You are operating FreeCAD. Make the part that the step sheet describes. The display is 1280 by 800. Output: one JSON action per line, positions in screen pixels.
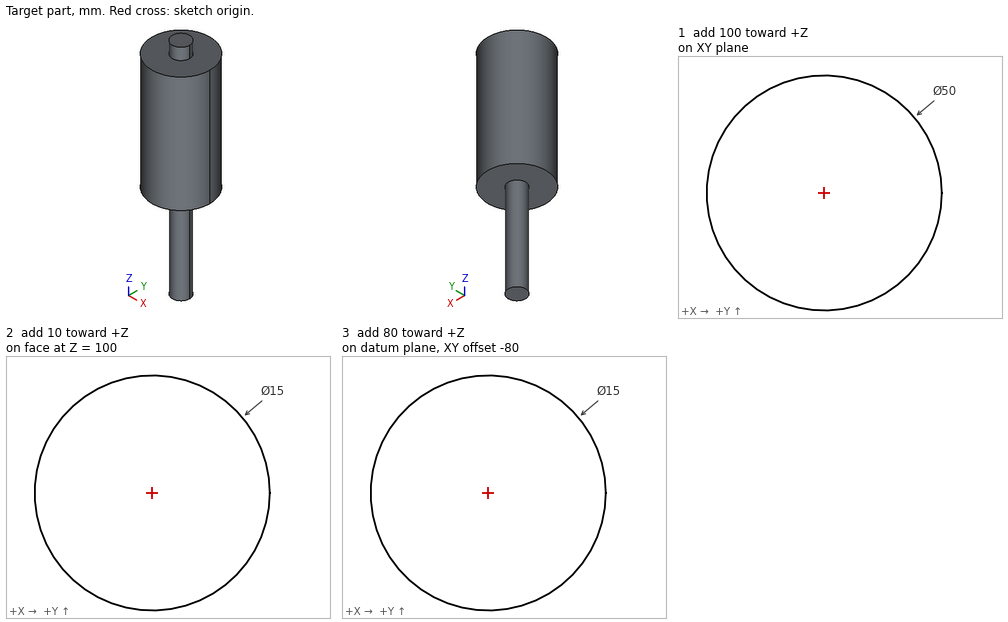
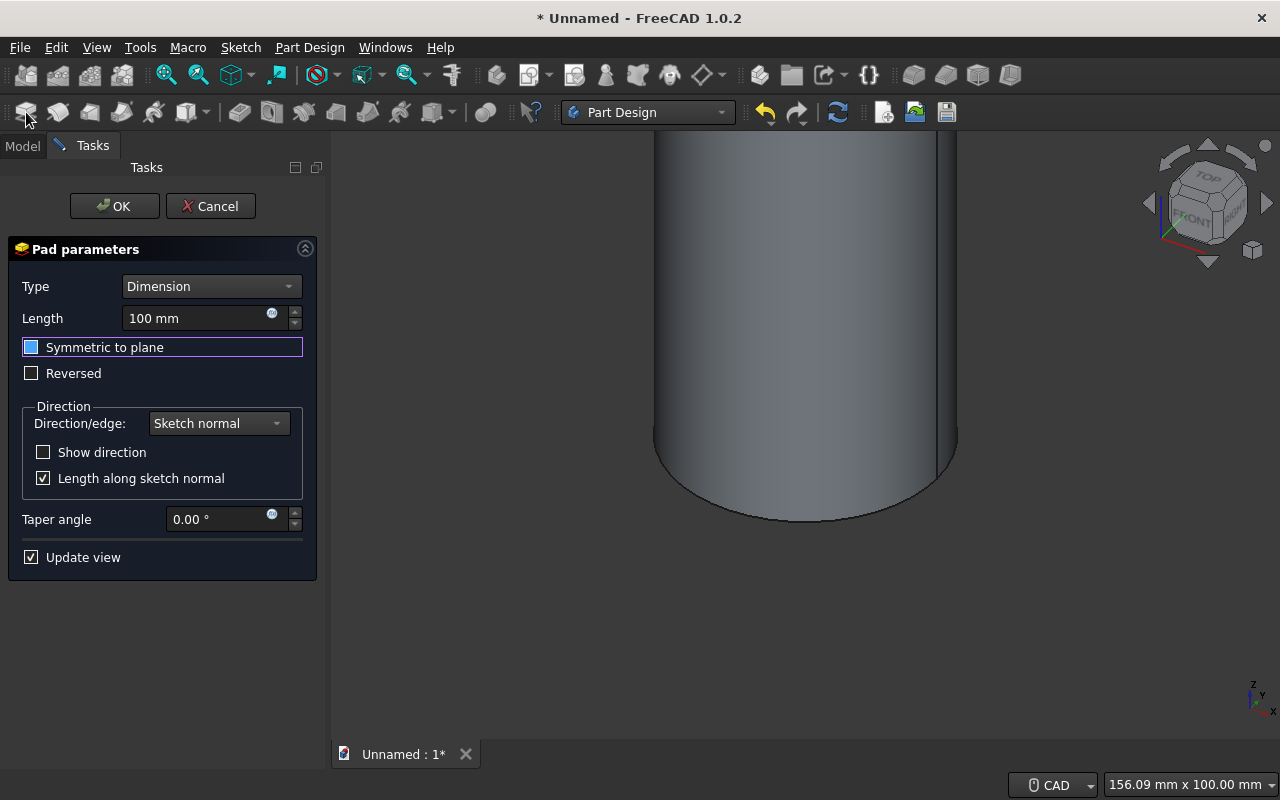
{"action": "left_click", "coordinate": [115, 206]}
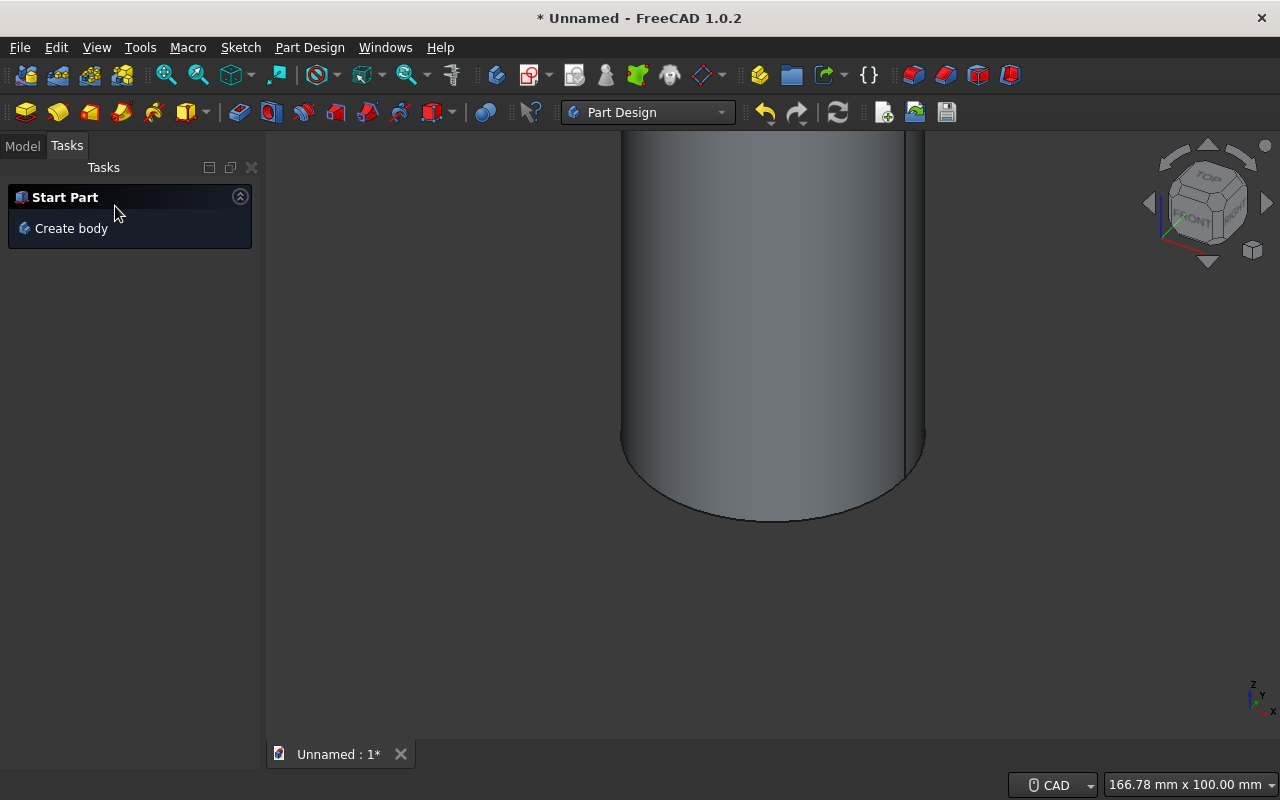
{"action": "left_click", "coordinate": [168, 76]}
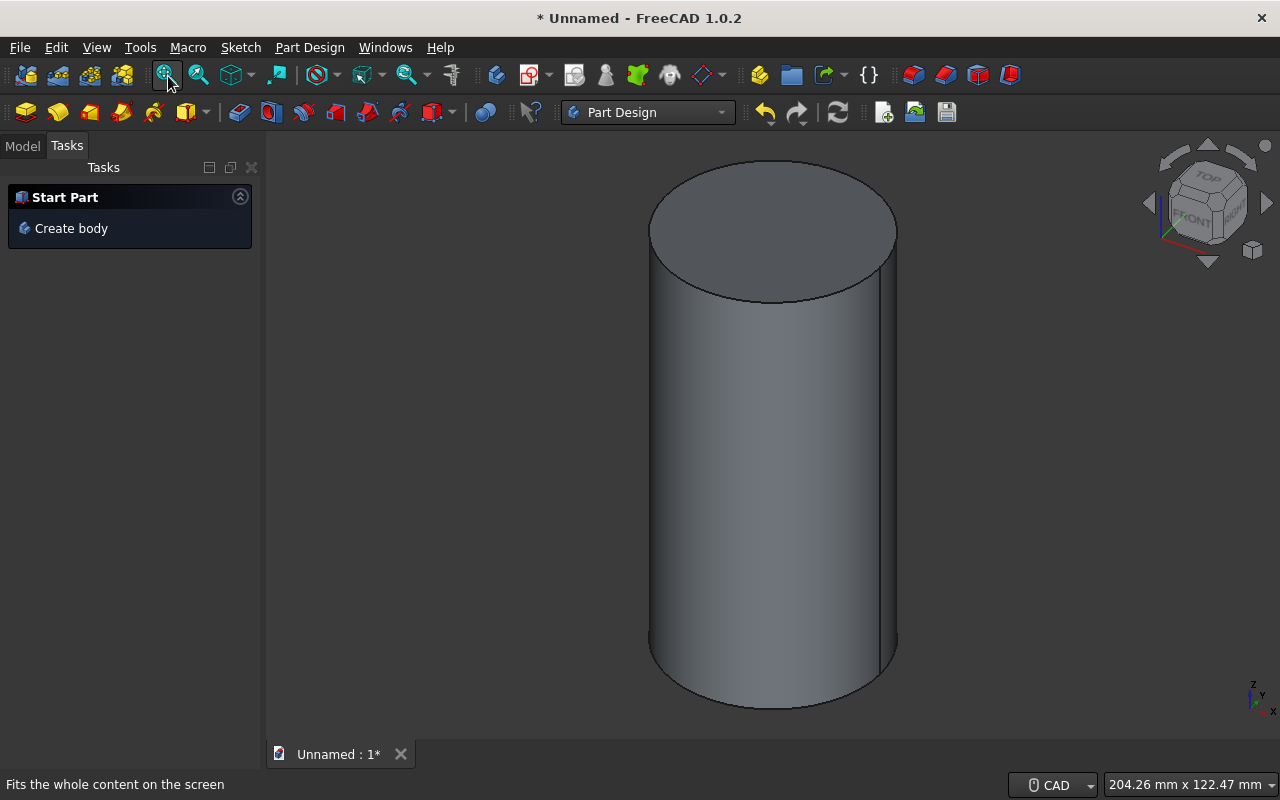
{"action": "left_click", "coordinate": [773, 231]}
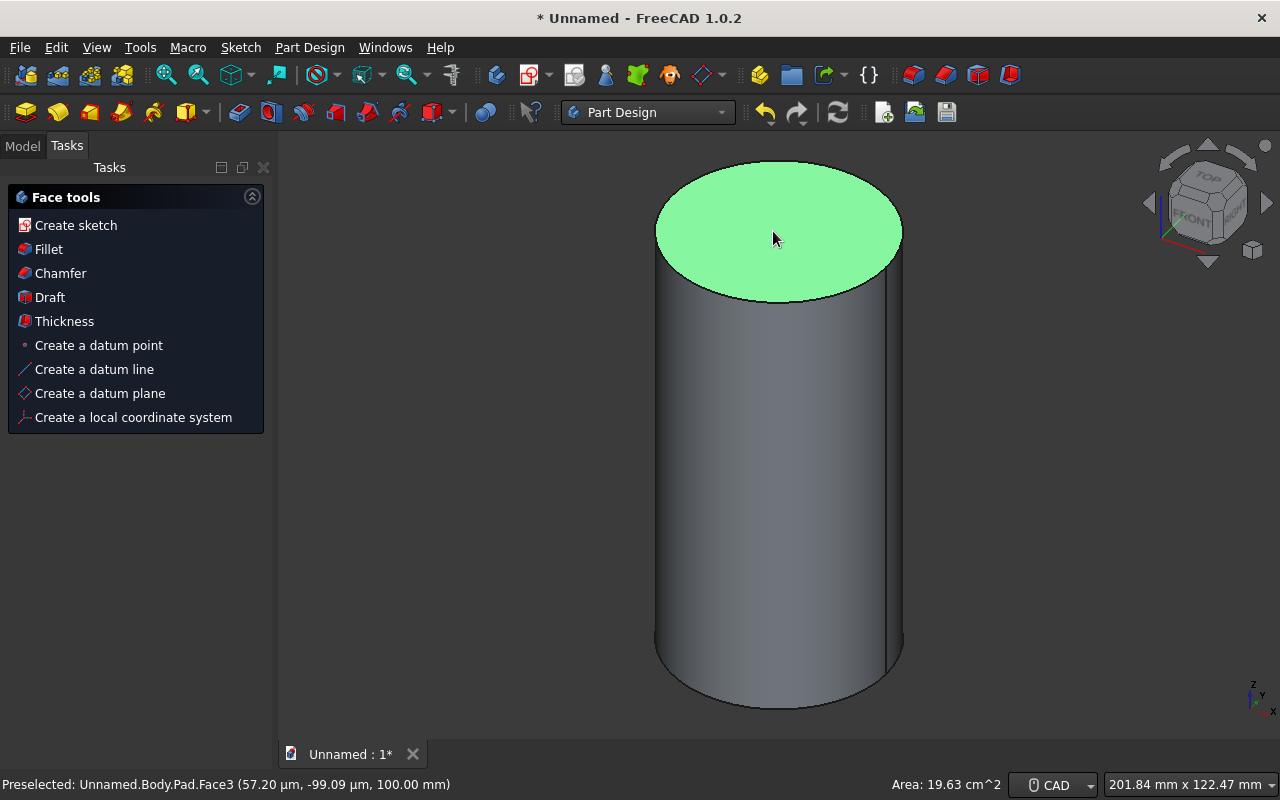
{"action": "left_click", "coordinate": [530, 76]}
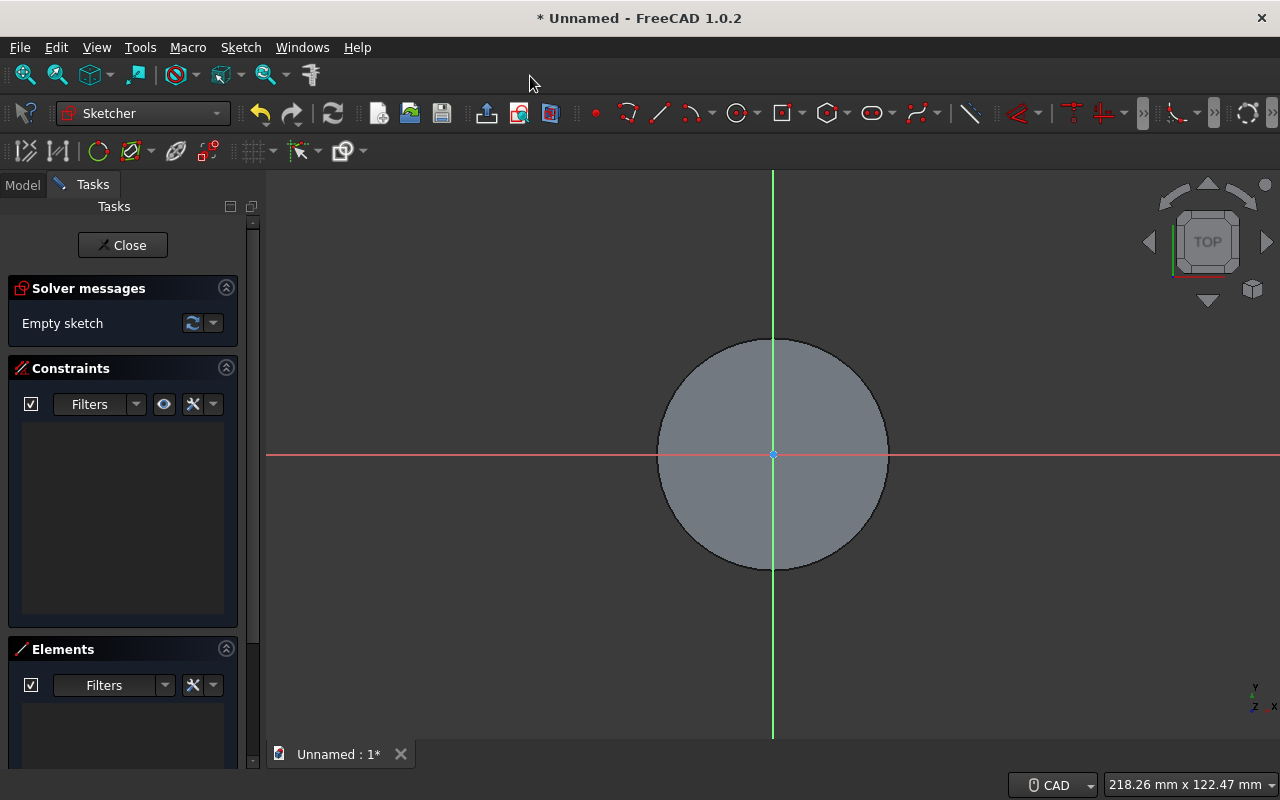
{"action": "scroll", "coordinate": [790, 454], "scroll_direction": "up", "scroll_amount": 8}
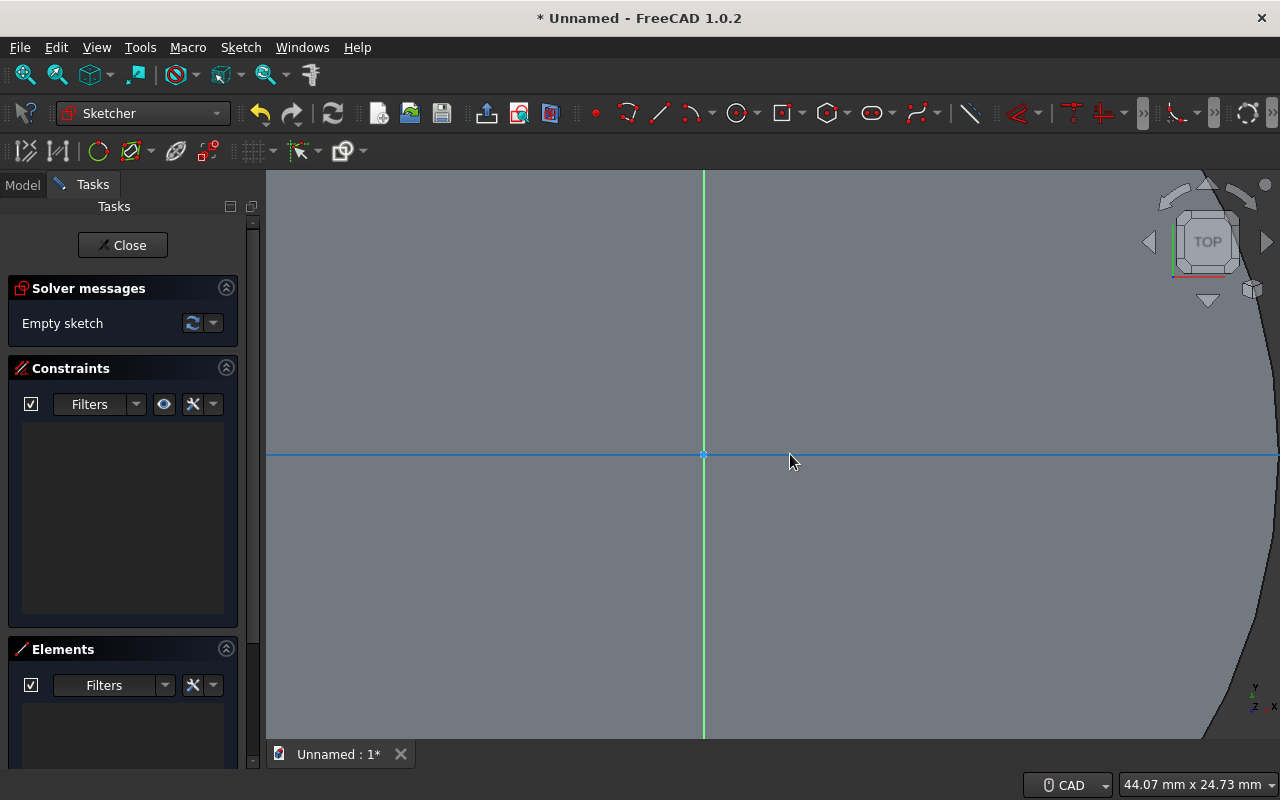
{"action": "left_click", "coordinate": [738, 114]}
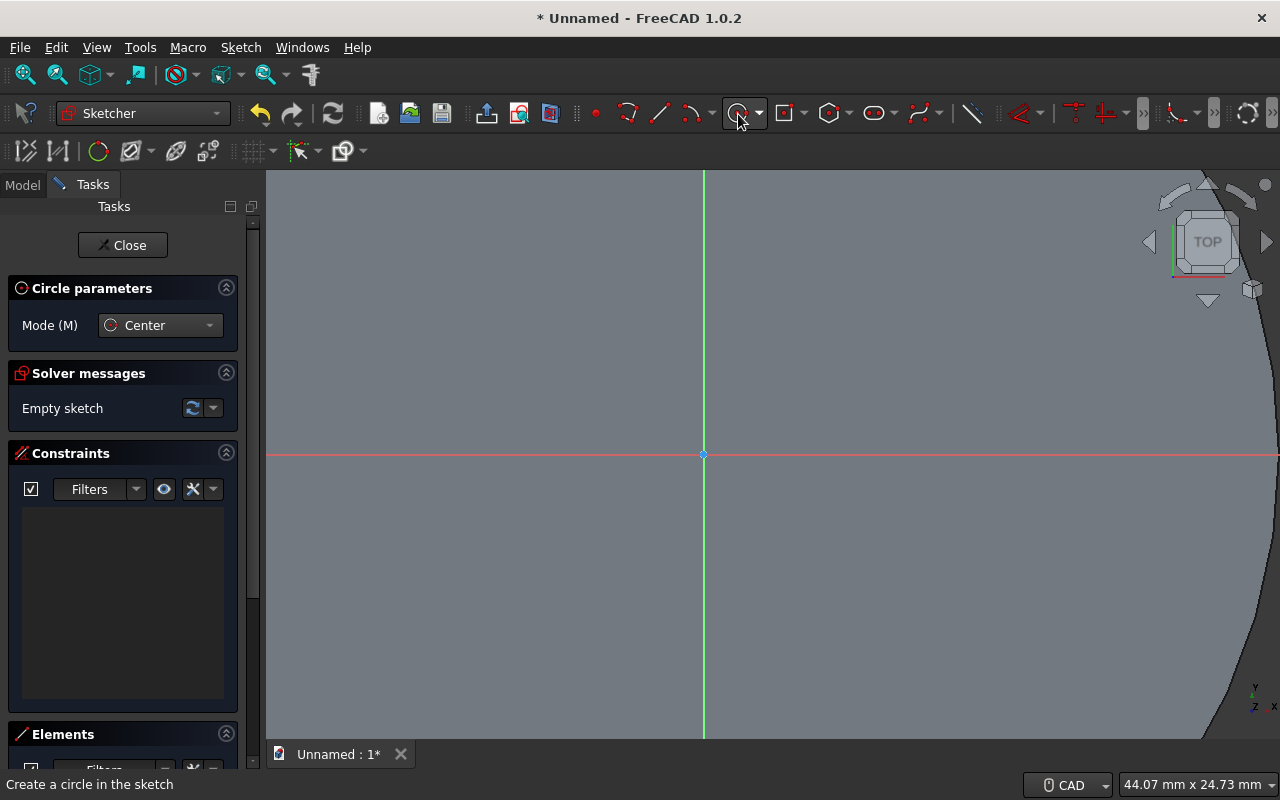
{"action": "left_click", "coordinate": [704, 454]}
{"action": "mouse_move", "coordinate": [826, 332]}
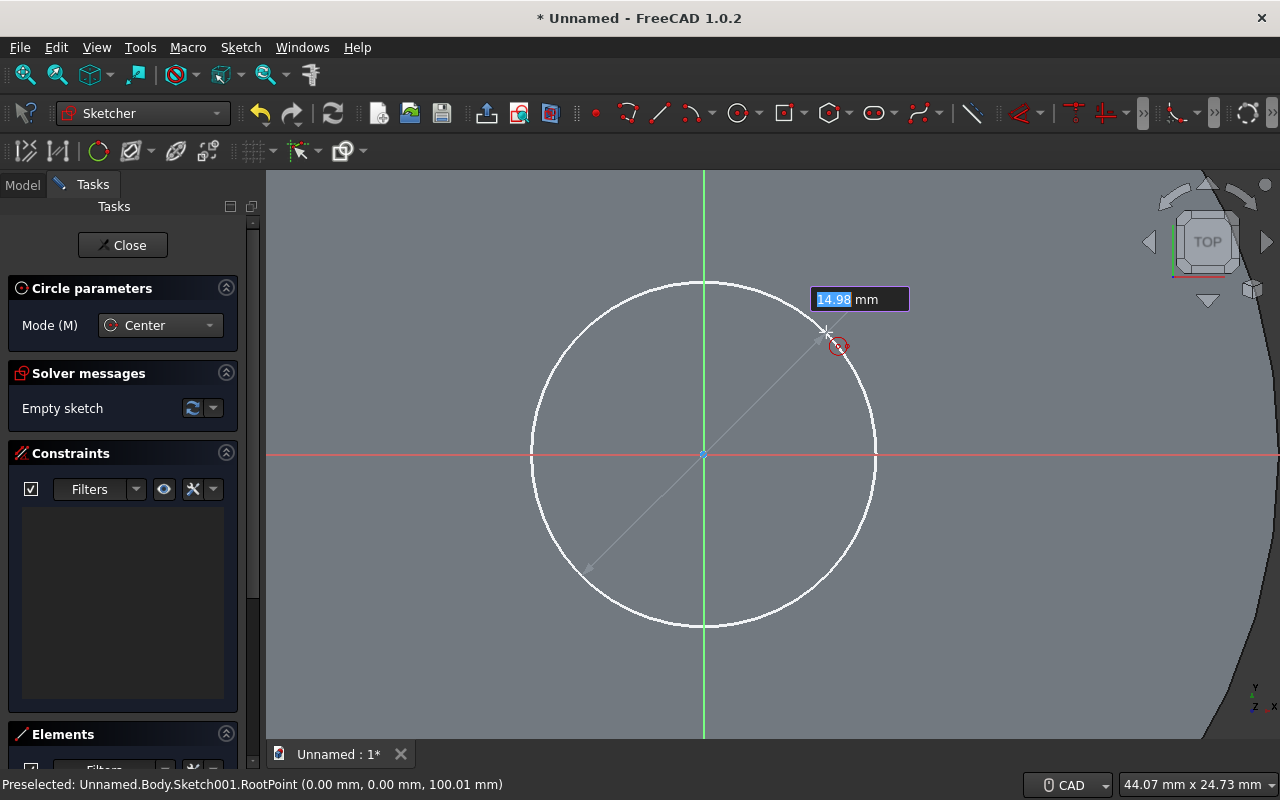
{"action": "type", "text": "15"}
{"action": "key", "text": "Return"}
{"action": "key", "text": "Escape"}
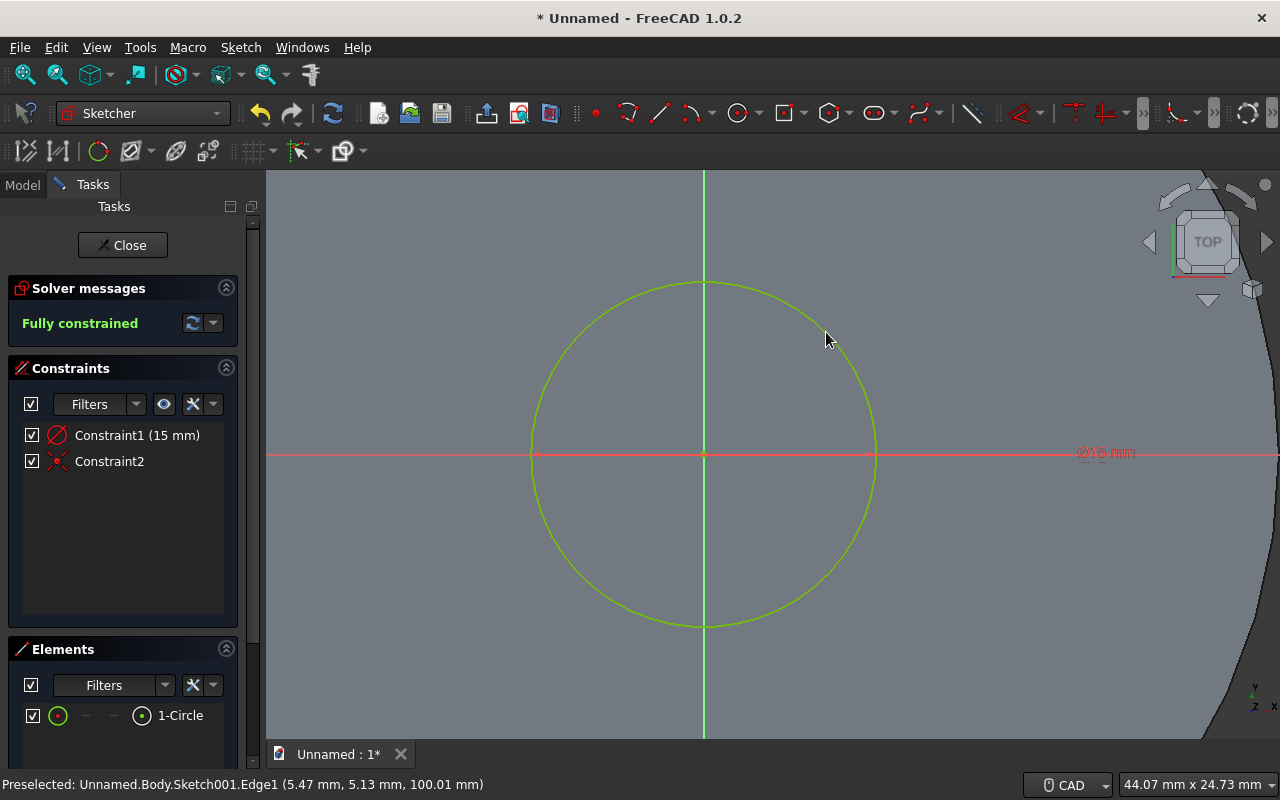
{"action": "left_click", "coordinate": [123, 245]}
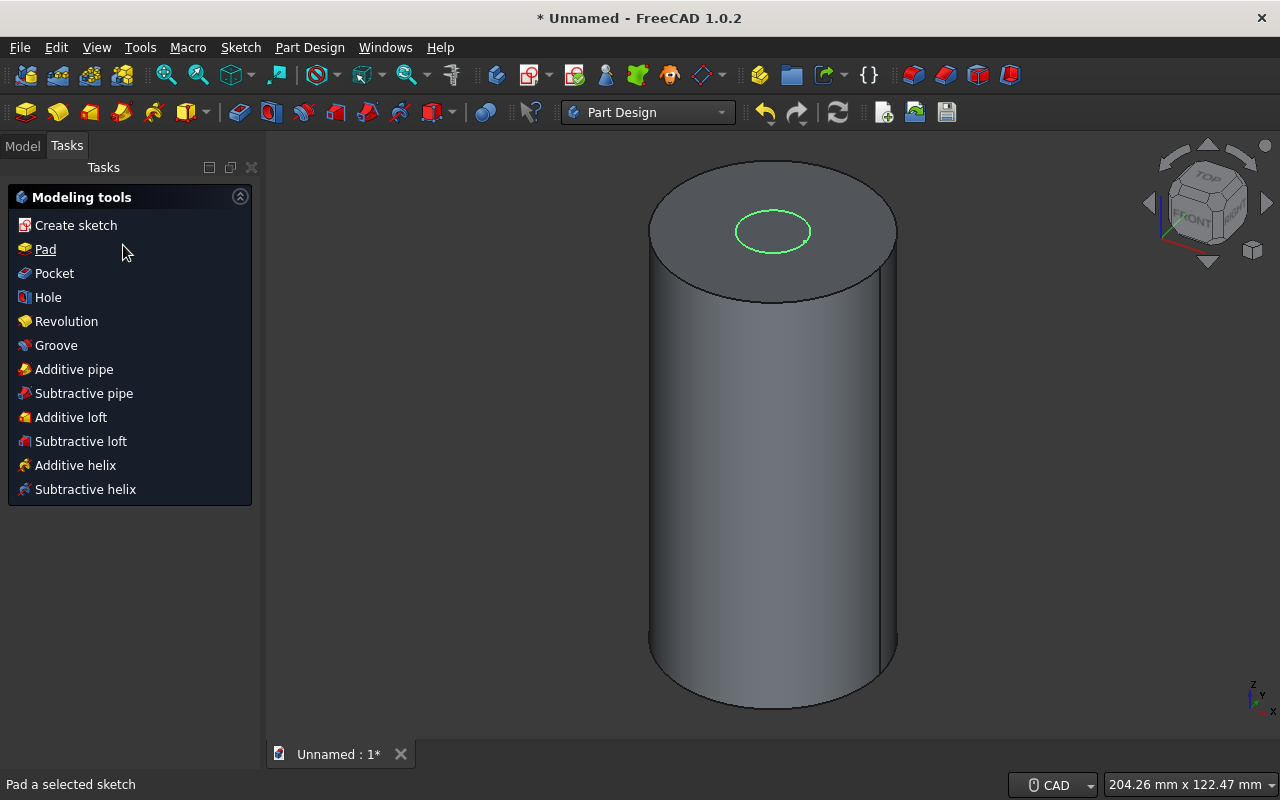
{"action": "left_click", "coordinate": [26, 112]}